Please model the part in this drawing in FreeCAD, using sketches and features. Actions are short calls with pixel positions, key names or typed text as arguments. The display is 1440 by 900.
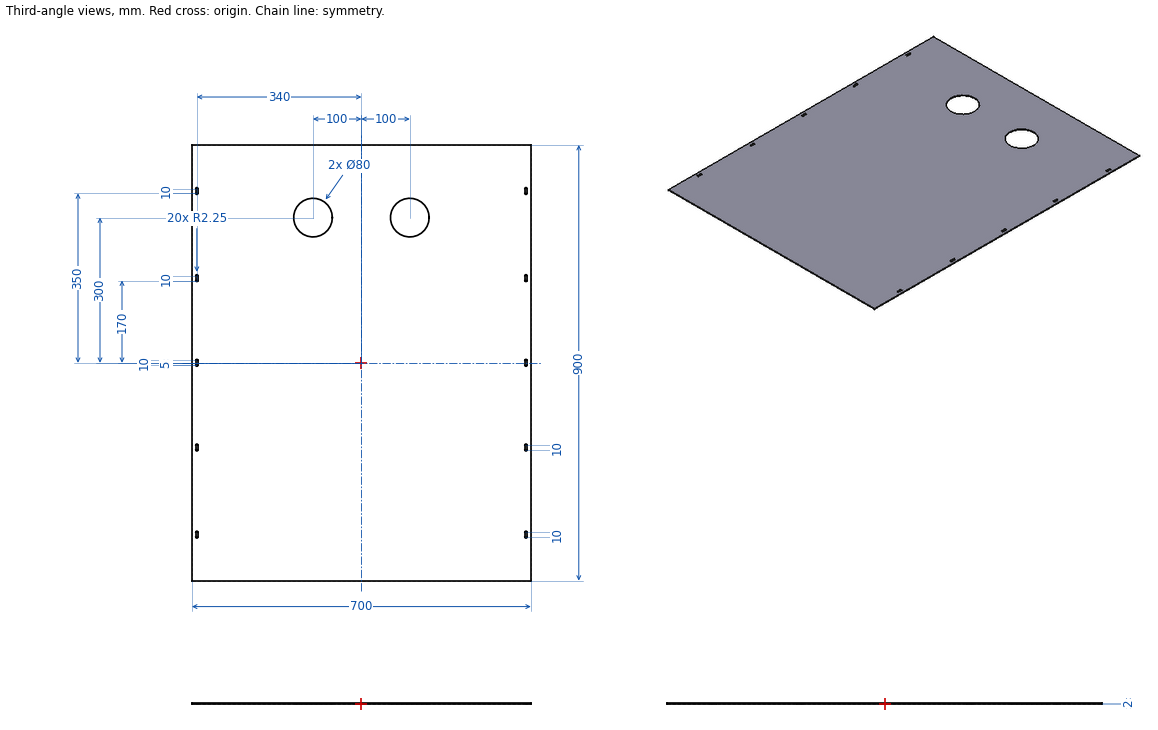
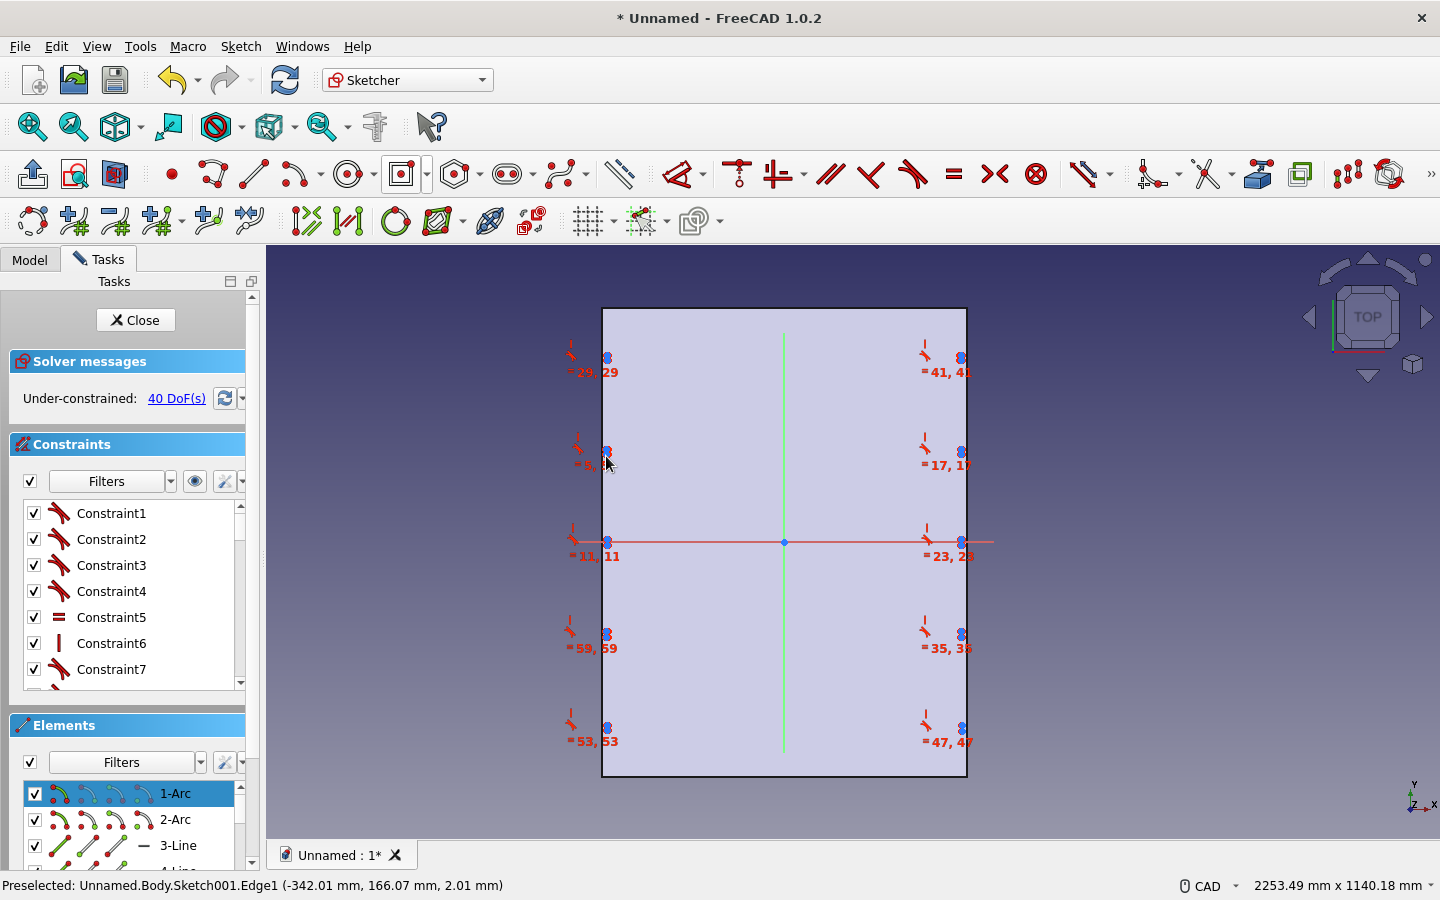
scroll(607, 546, up, 13)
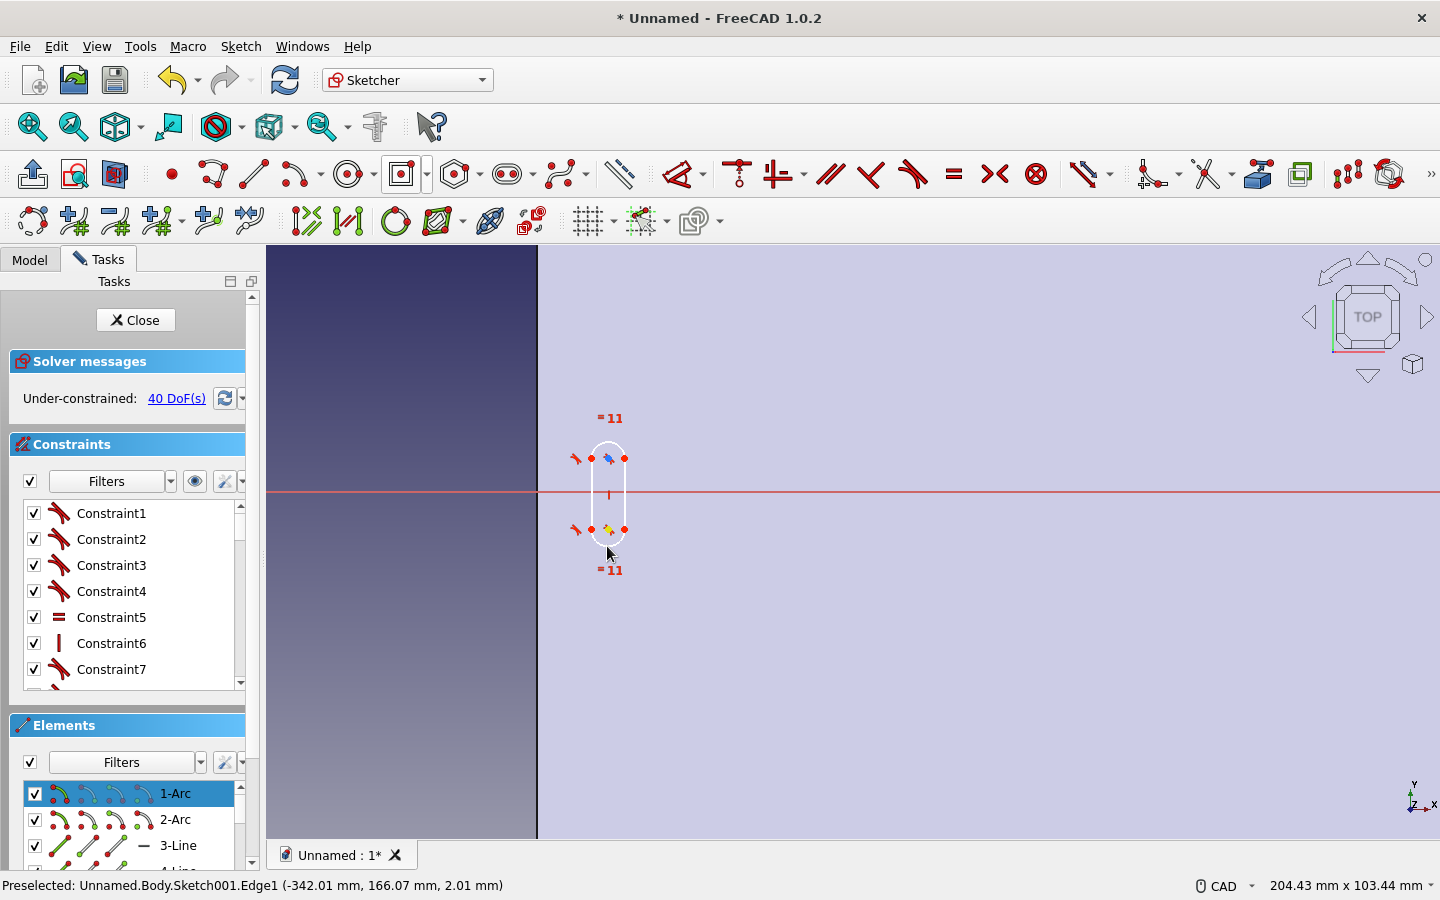
click(598, 543)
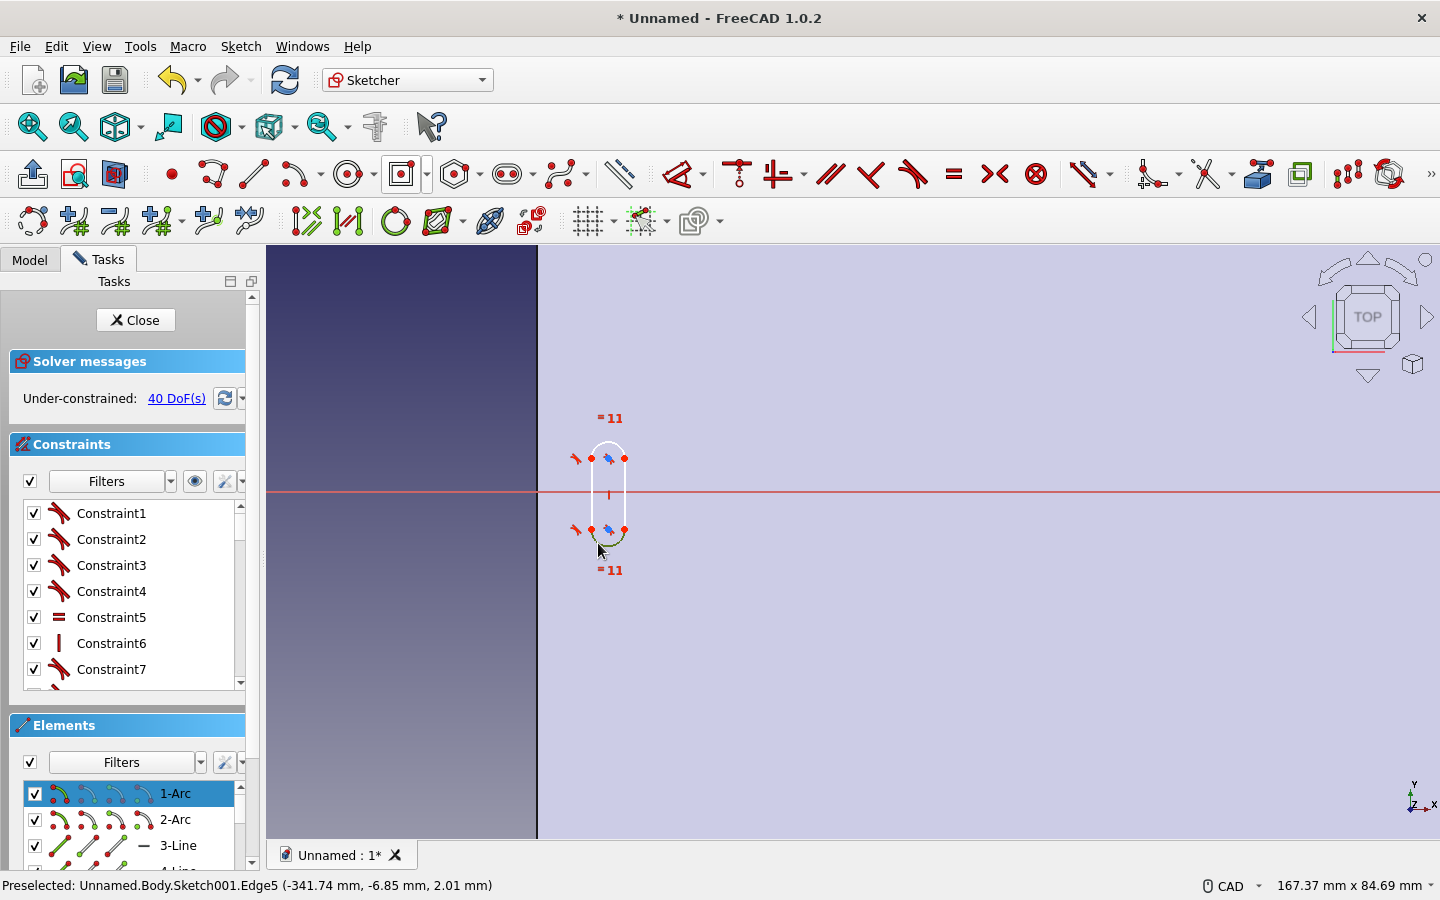
scroll(607, 546, down, 13)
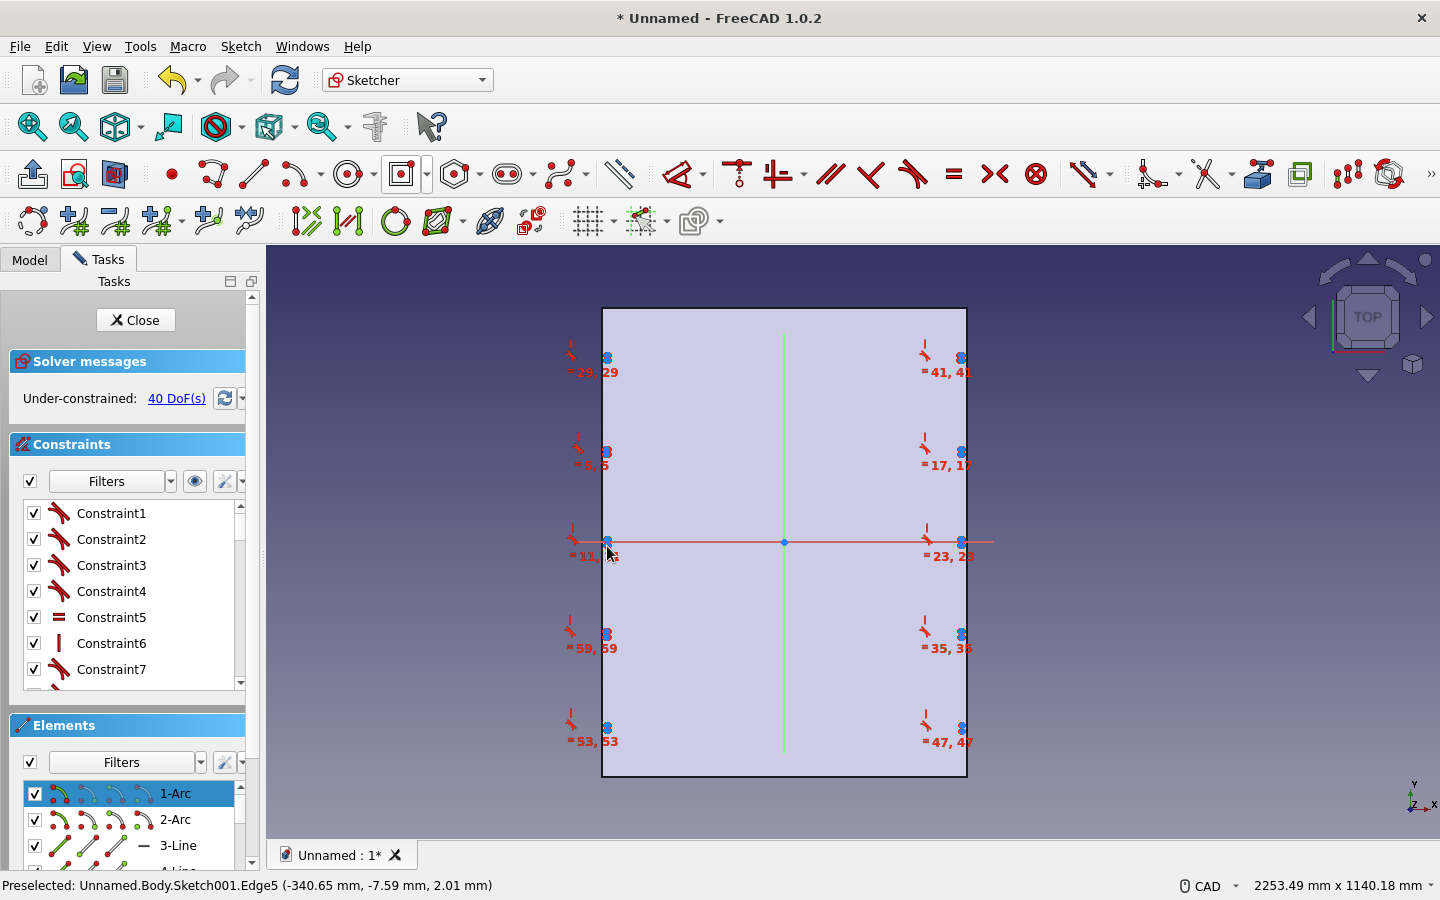
scroll(961, 456, up, 14)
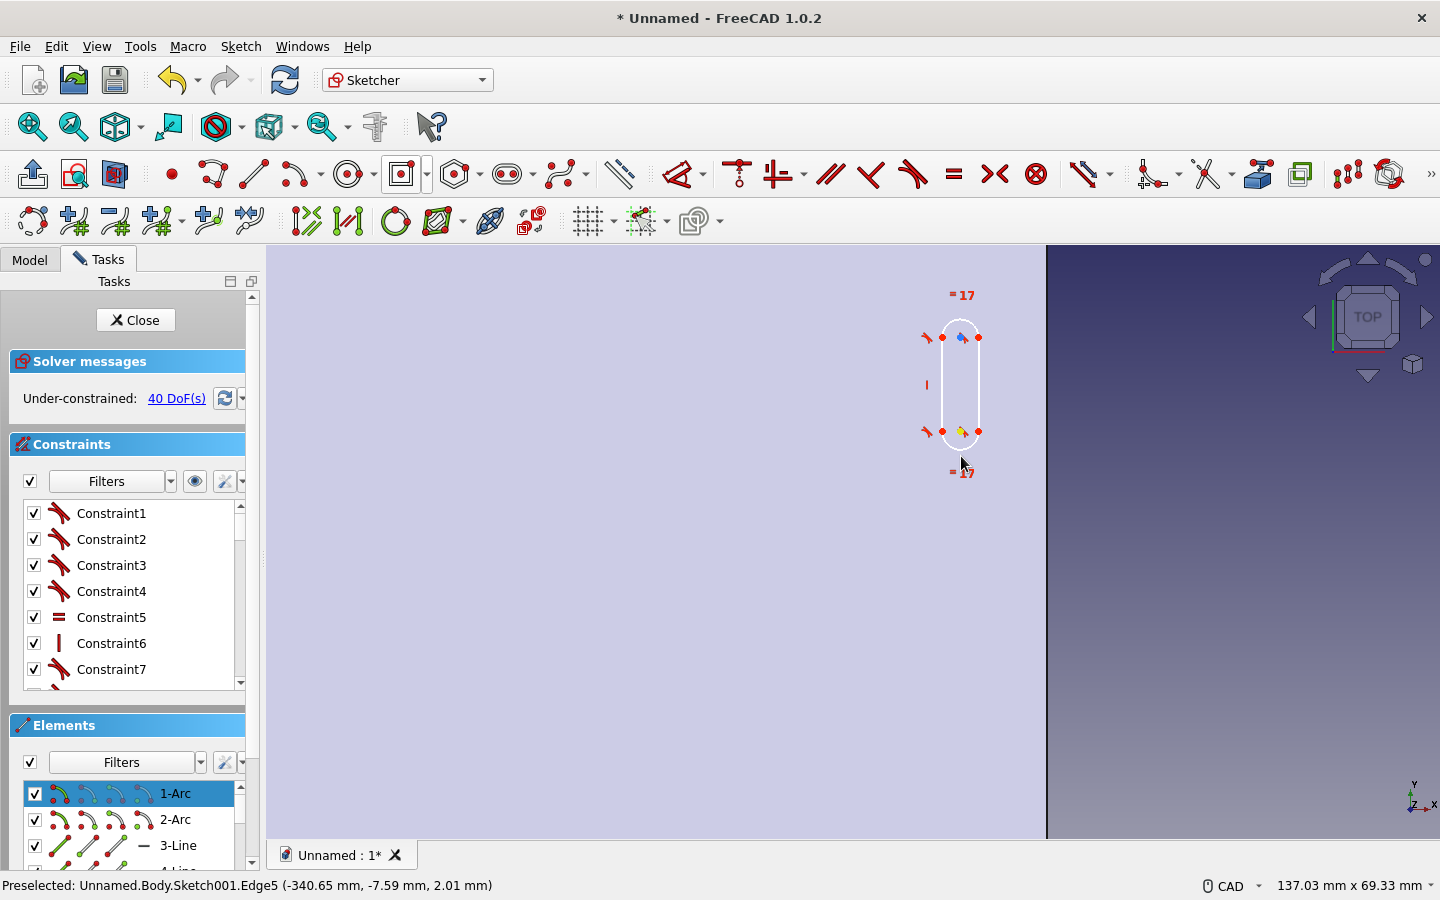
click(950, 446)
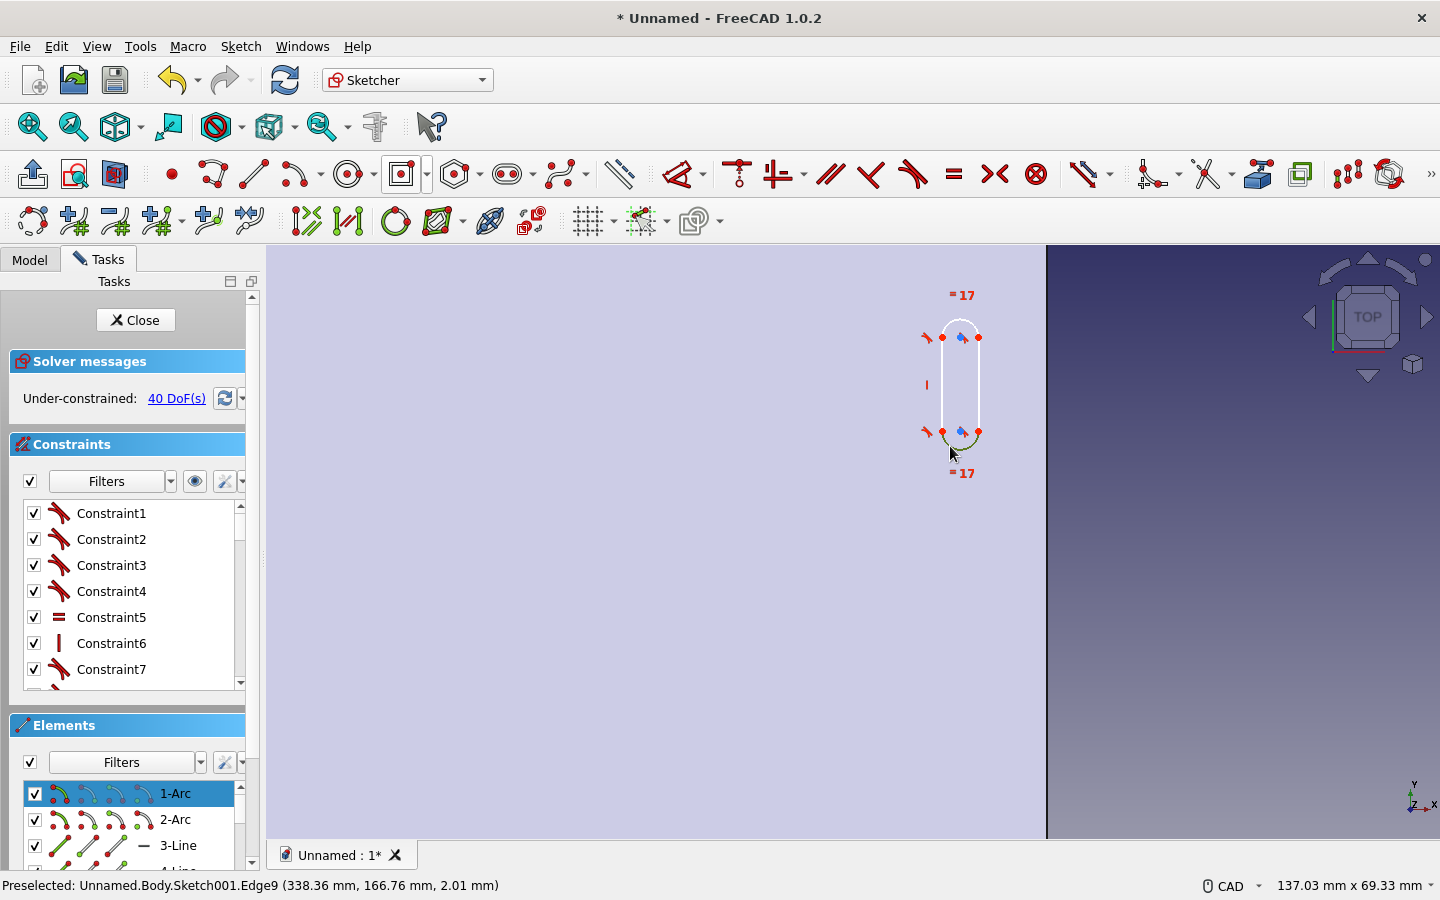
scroll(962, 456, down, 14)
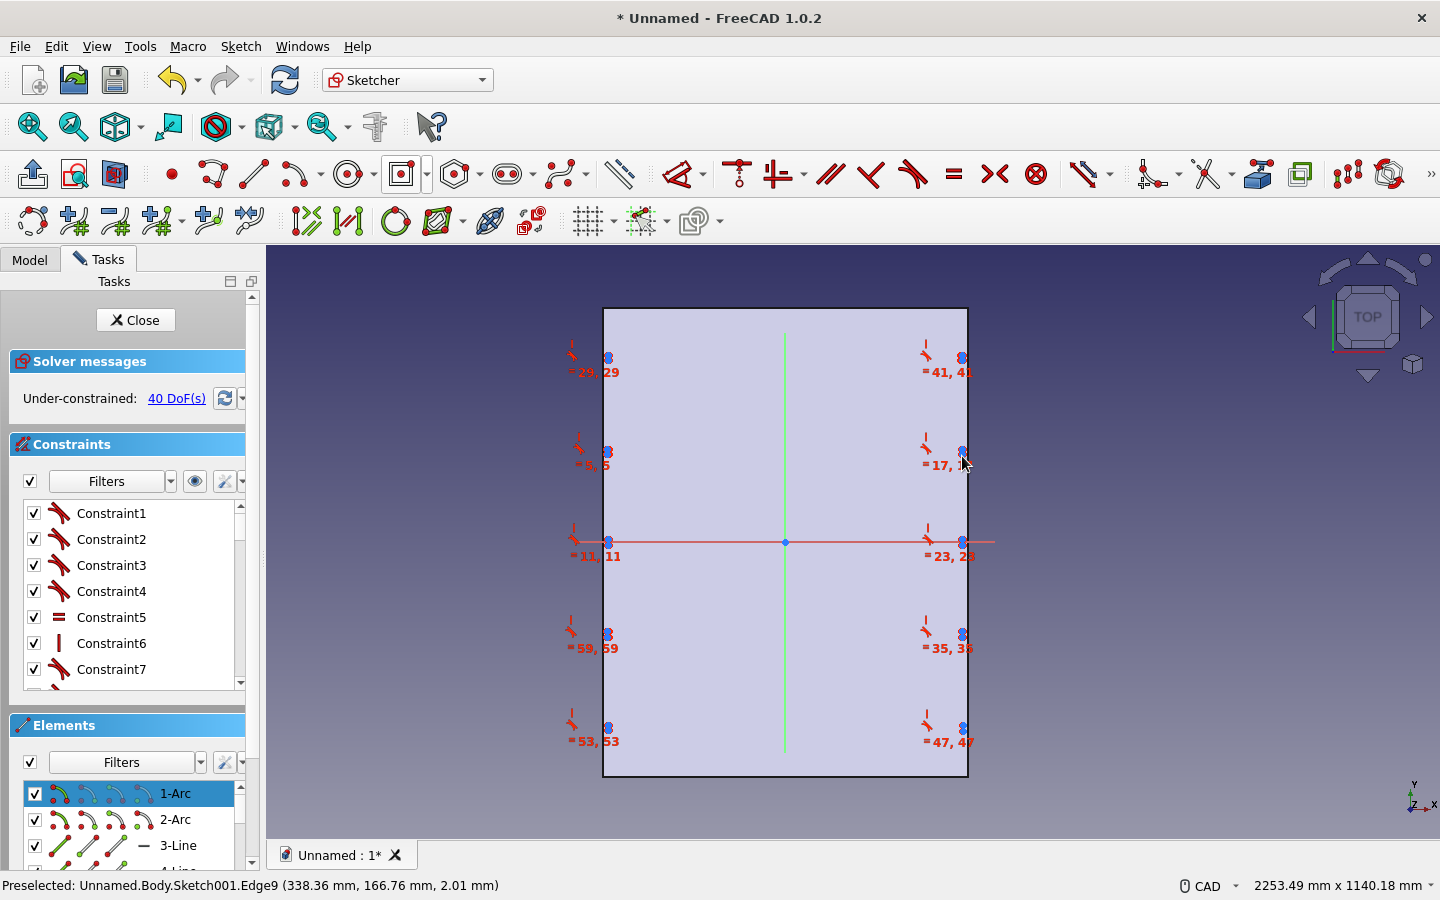
scroll(962, 546, up, 13)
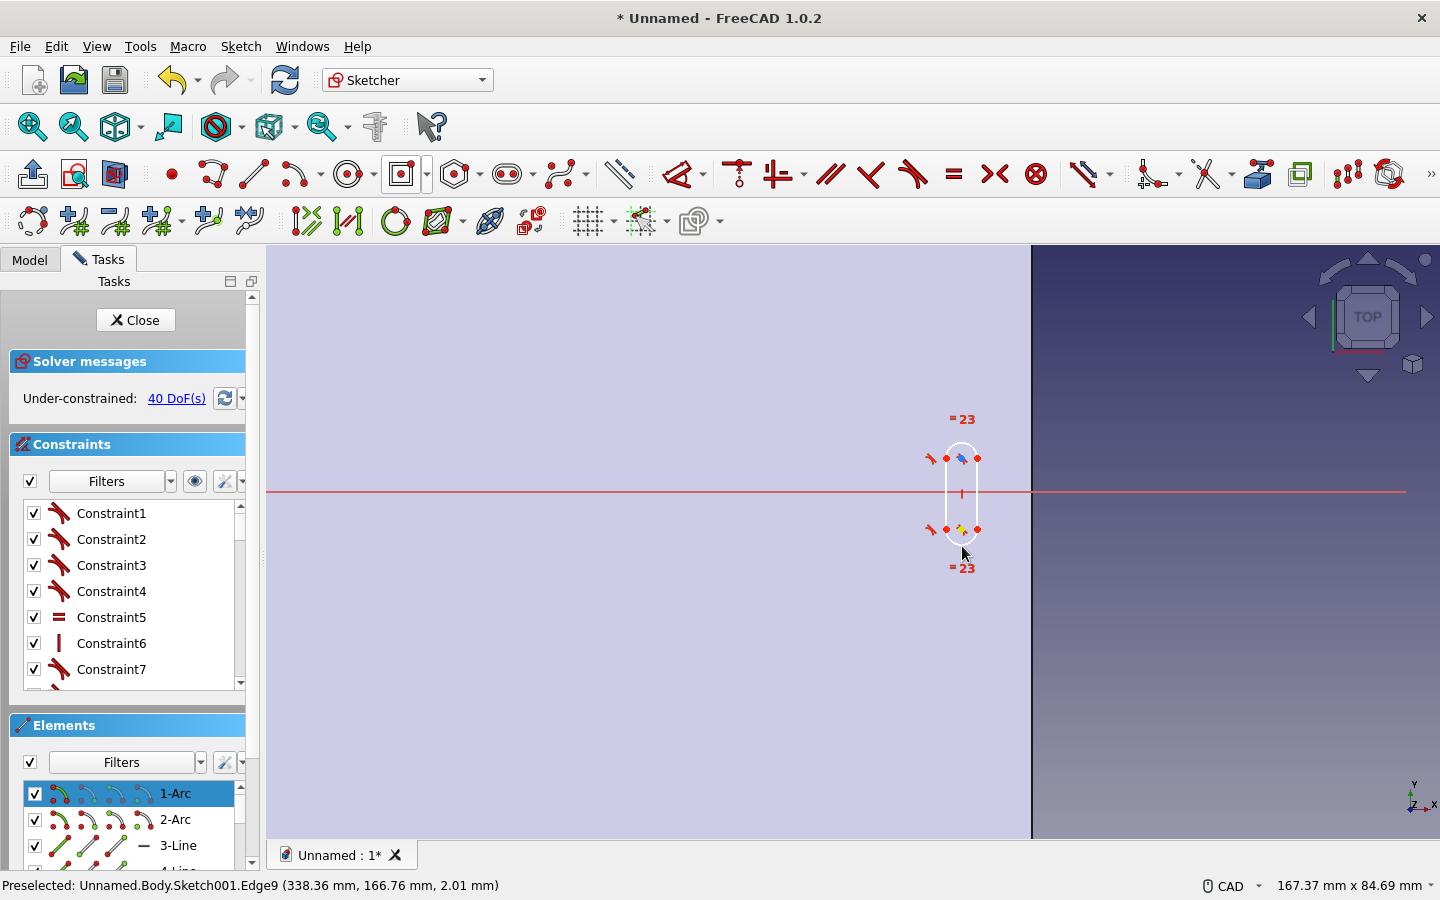
click(952, 542)